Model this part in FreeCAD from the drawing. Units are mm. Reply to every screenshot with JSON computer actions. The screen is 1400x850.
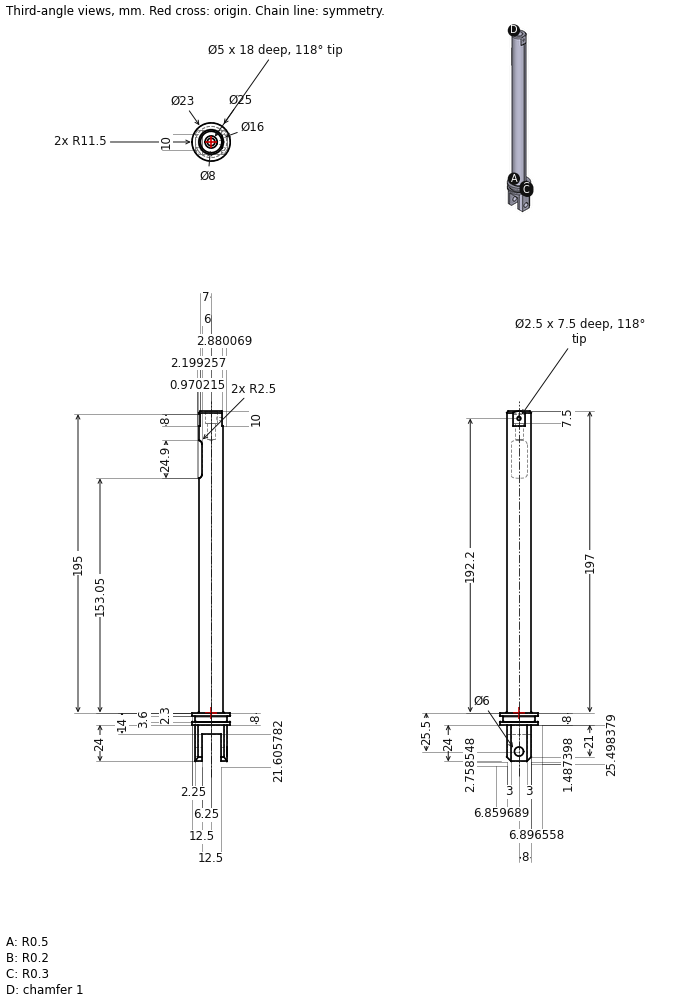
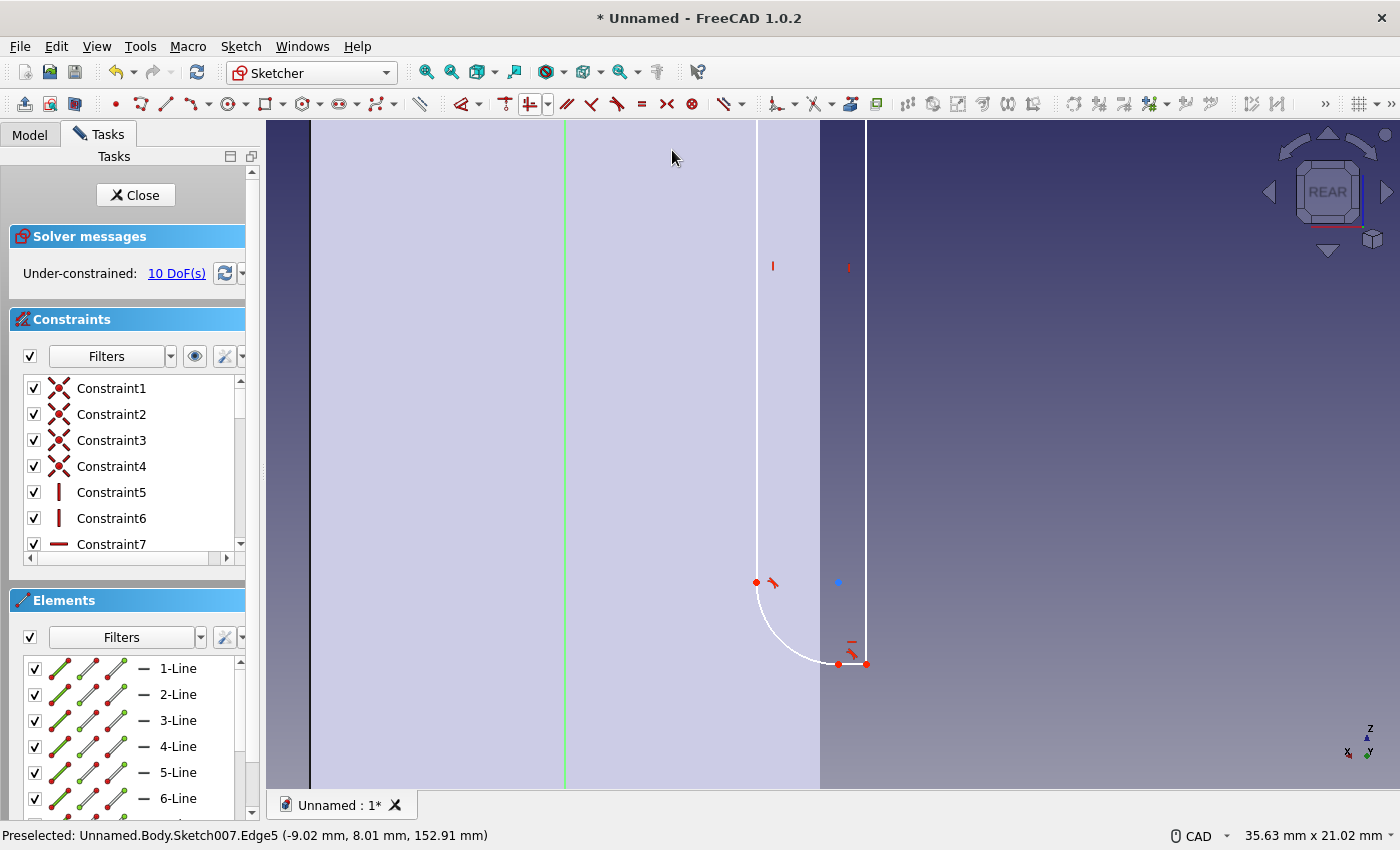
{"action": "scroll", "coordinate": [853, 667], "scroll_direction": "down", "scroll_amount": 6}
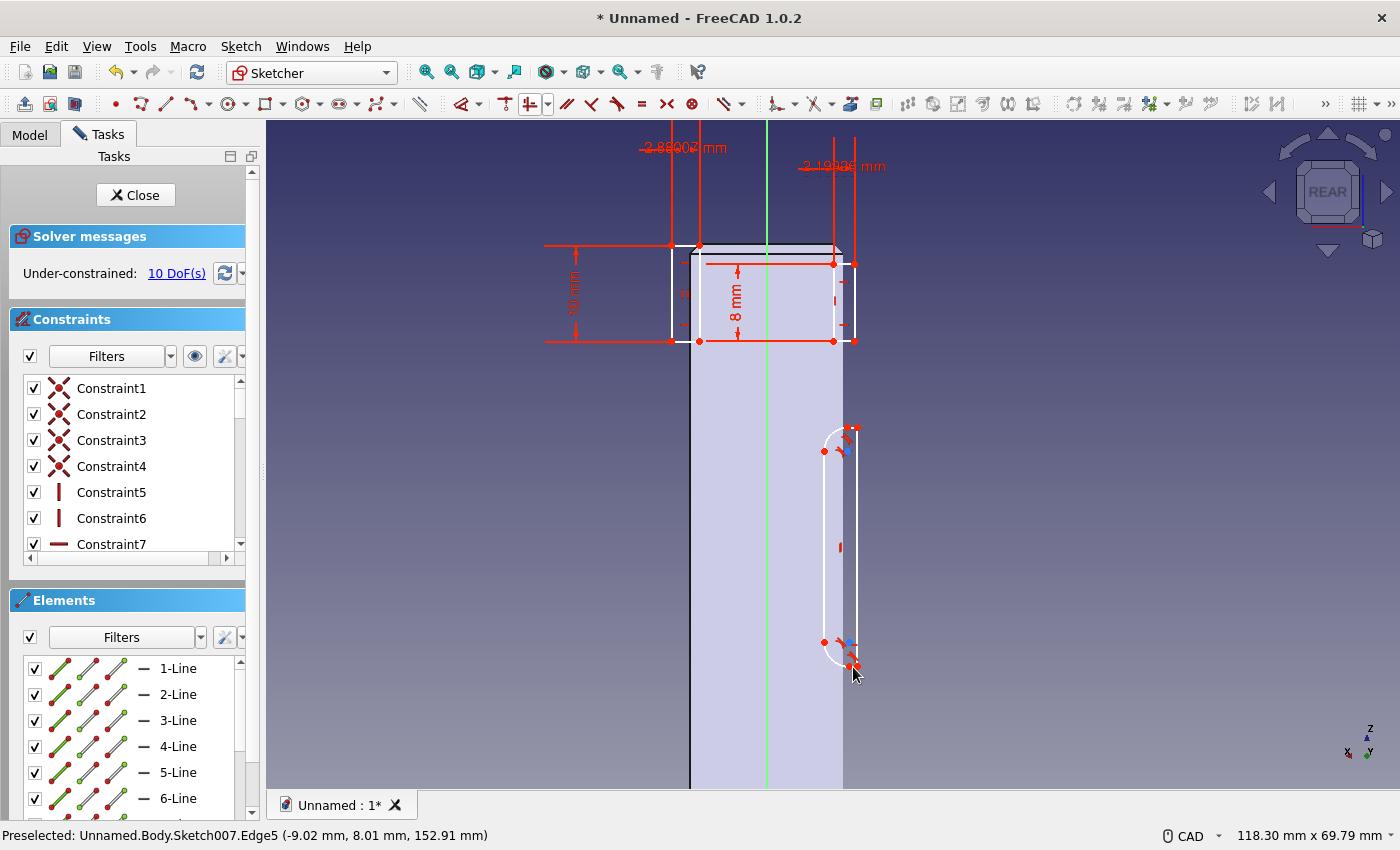
{"action": "scroll", "coordinate": [837, 430], "scroll_direction": "up", "scroll_amount": 2}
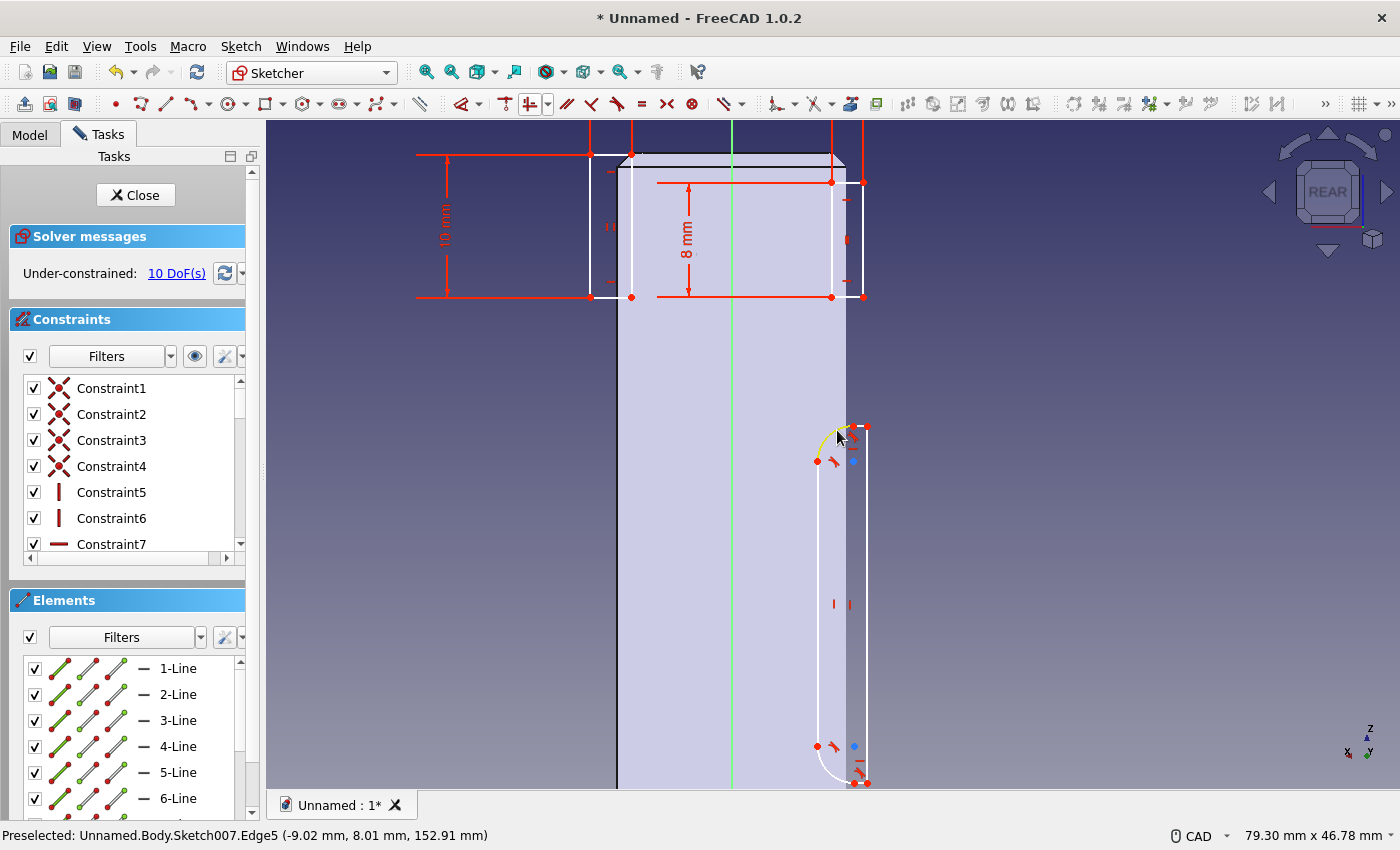
{"action": "left_click", "coordinate": [837, 430]}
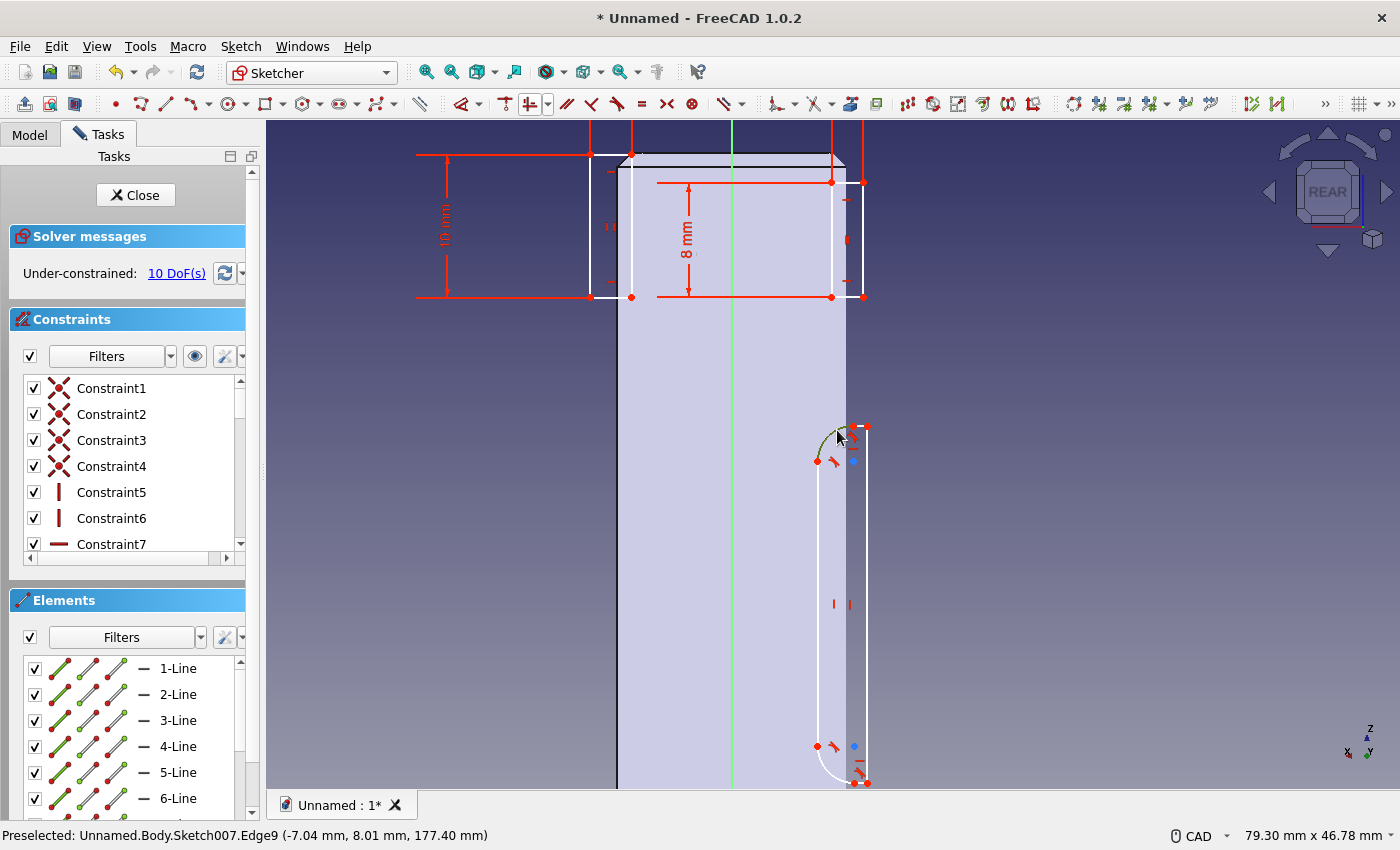
{"action": "left_click", "coordinate": [820, 758]}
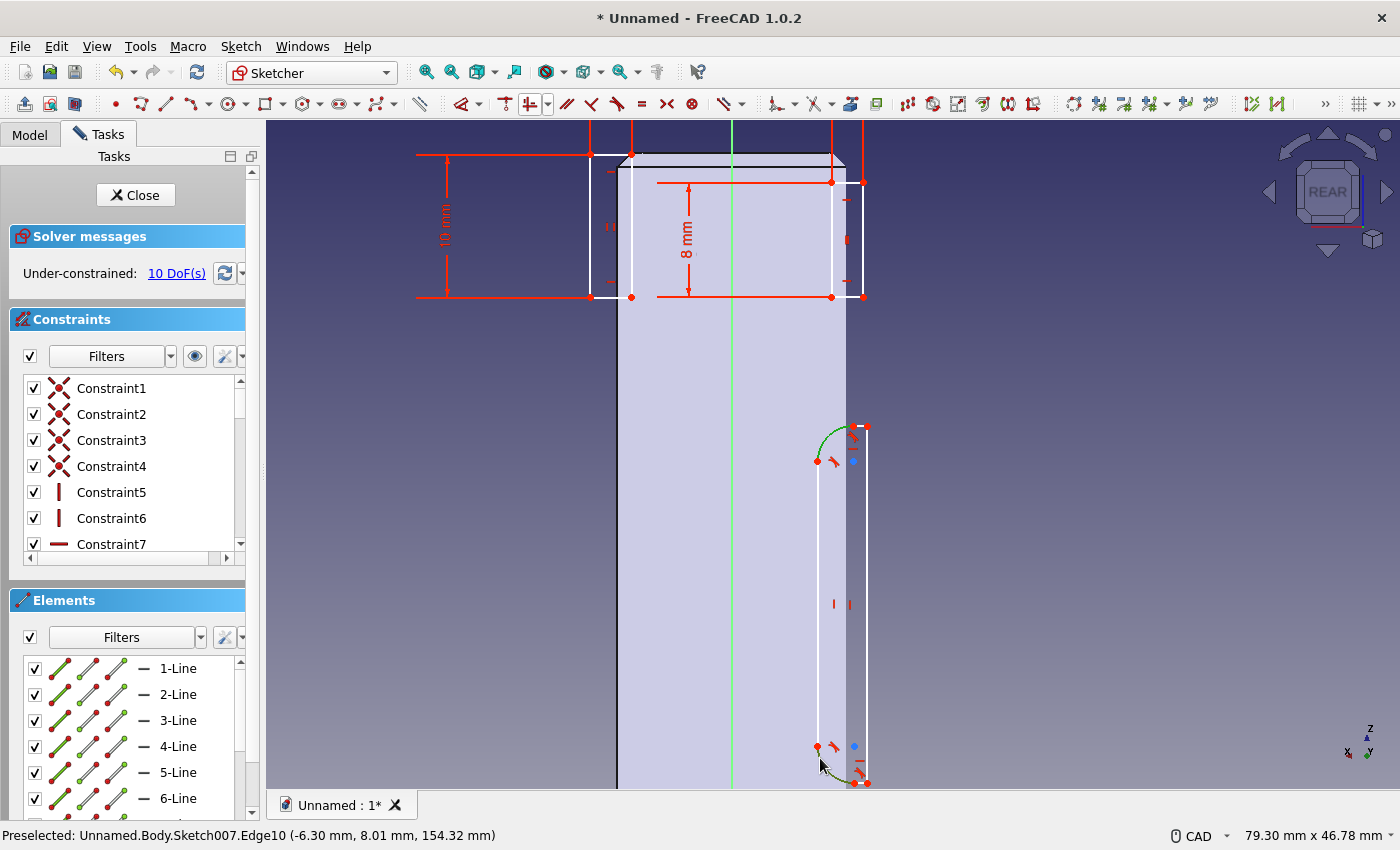
{"action": "left_click", "coordinate": [642, 104]}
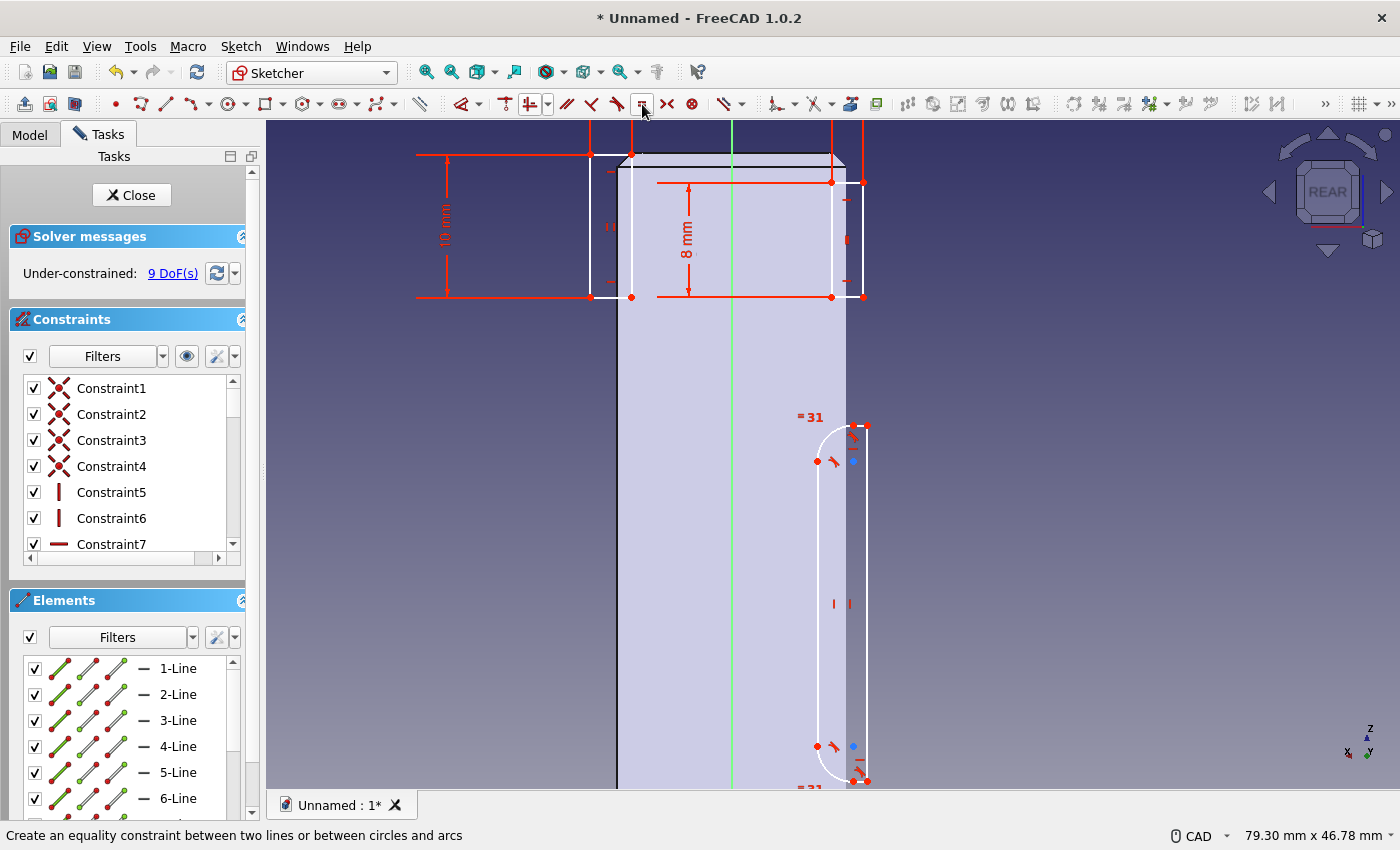
{"action": "left_click", "coordinate": [832, 297]}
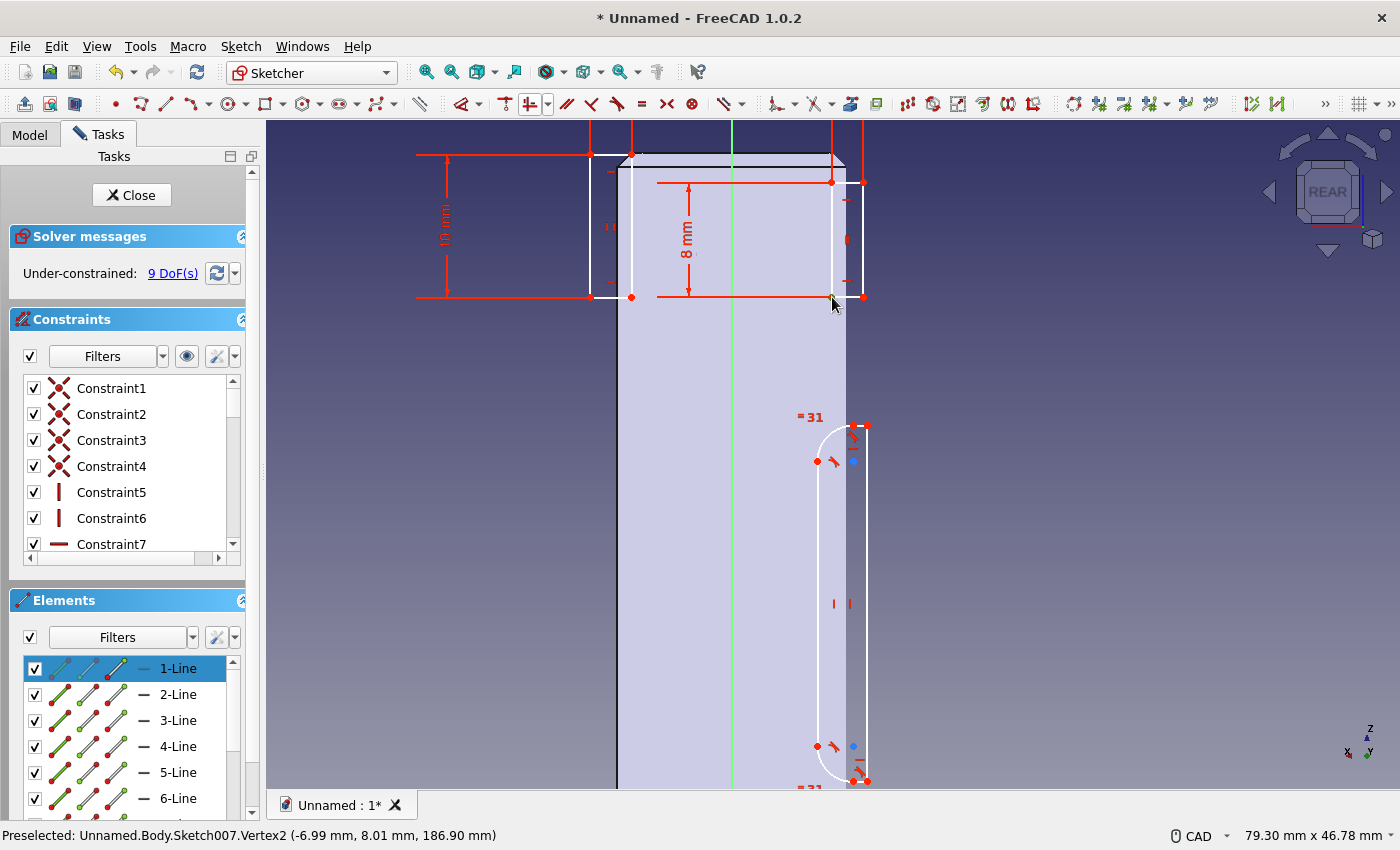
{"action": "left_click", "coordinate": [632, 298]}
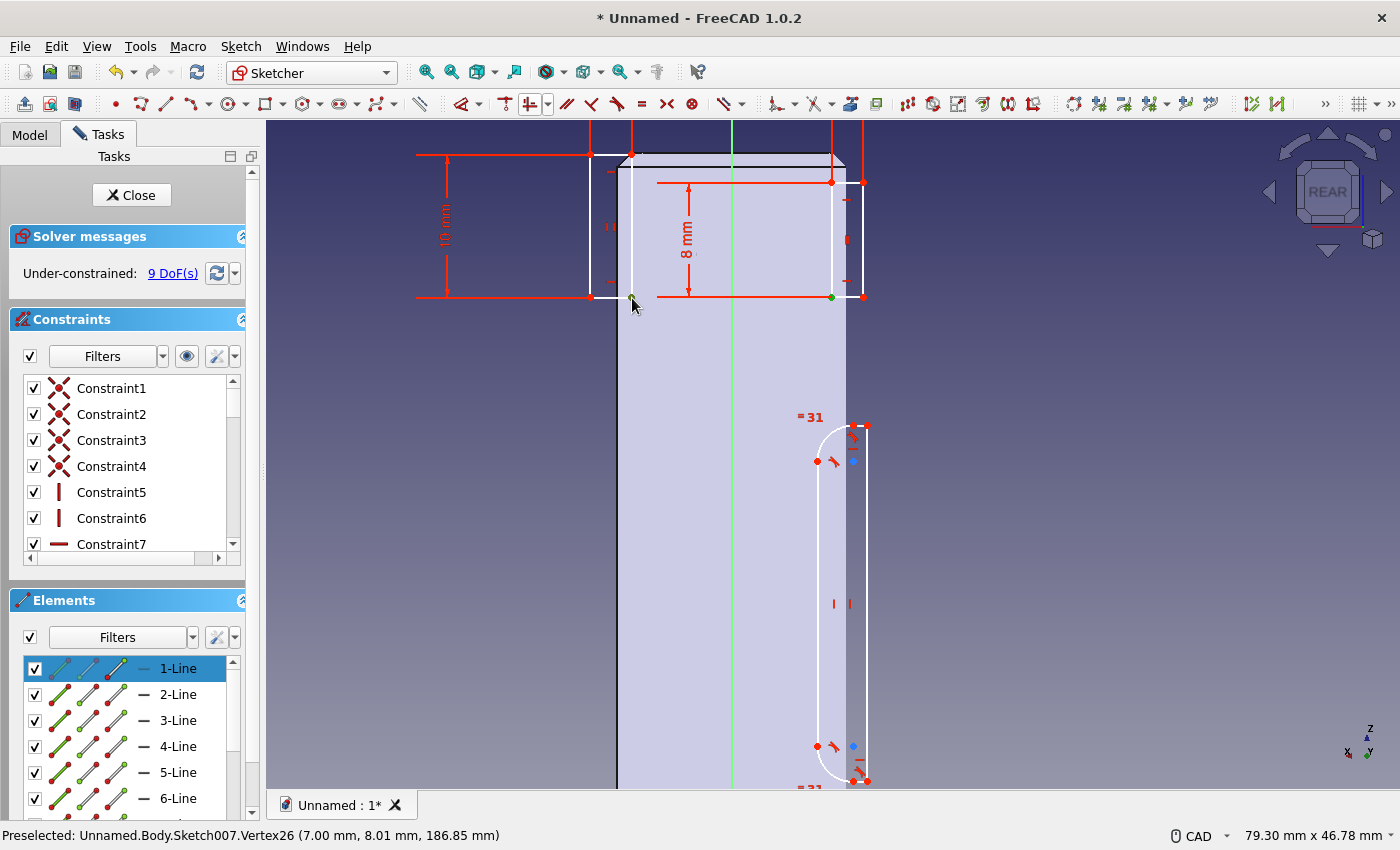
{"action": "left_click", "coordinate": [732, 717]}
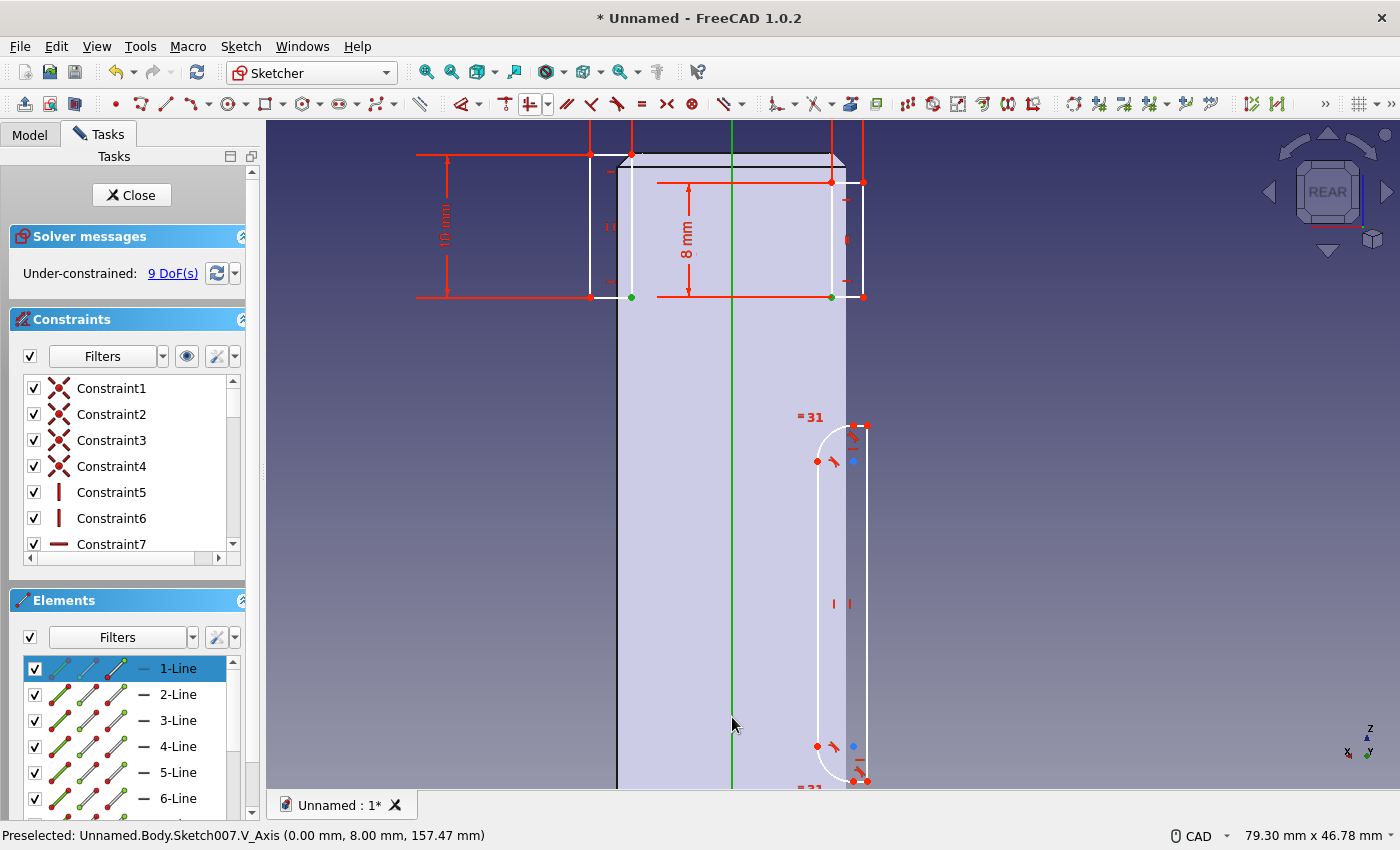
{"action": "left_click", "coordinate": [667, 104]}